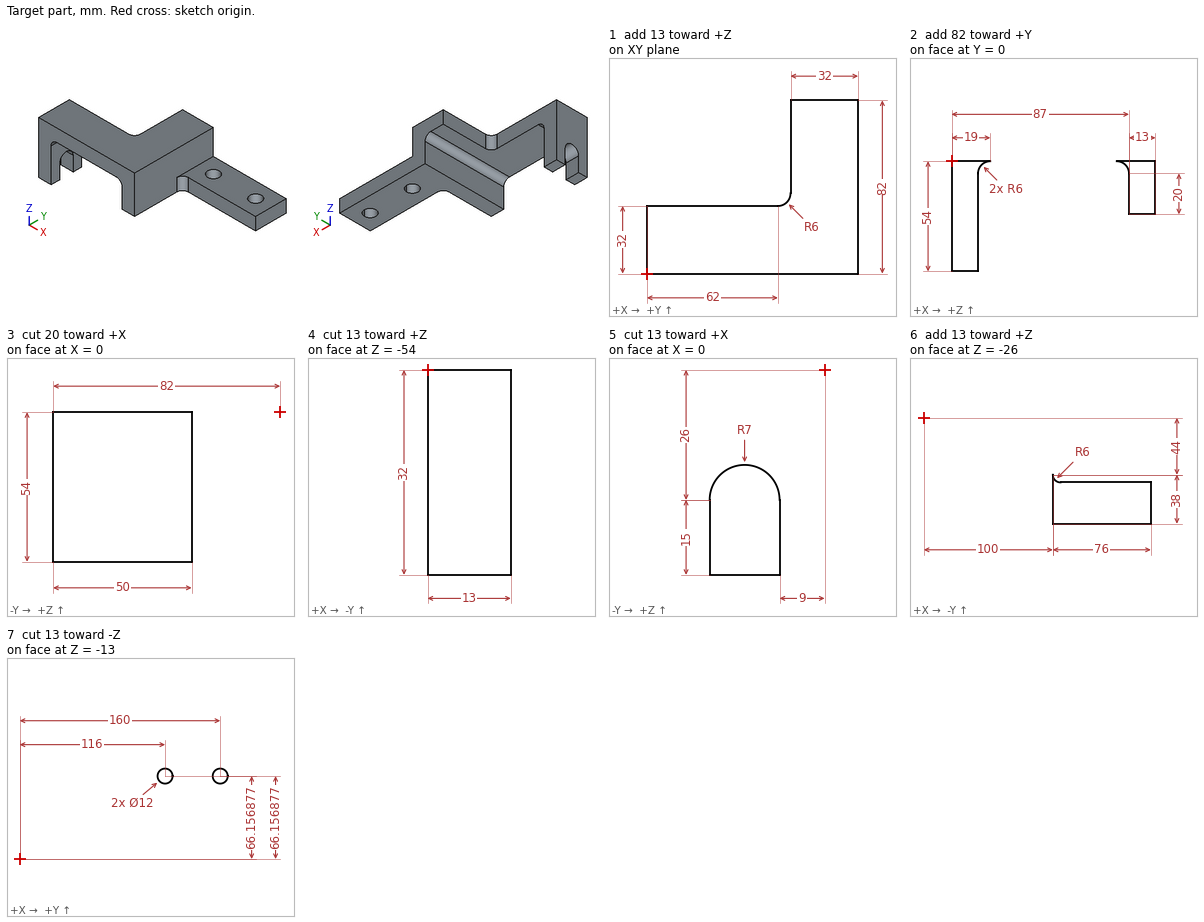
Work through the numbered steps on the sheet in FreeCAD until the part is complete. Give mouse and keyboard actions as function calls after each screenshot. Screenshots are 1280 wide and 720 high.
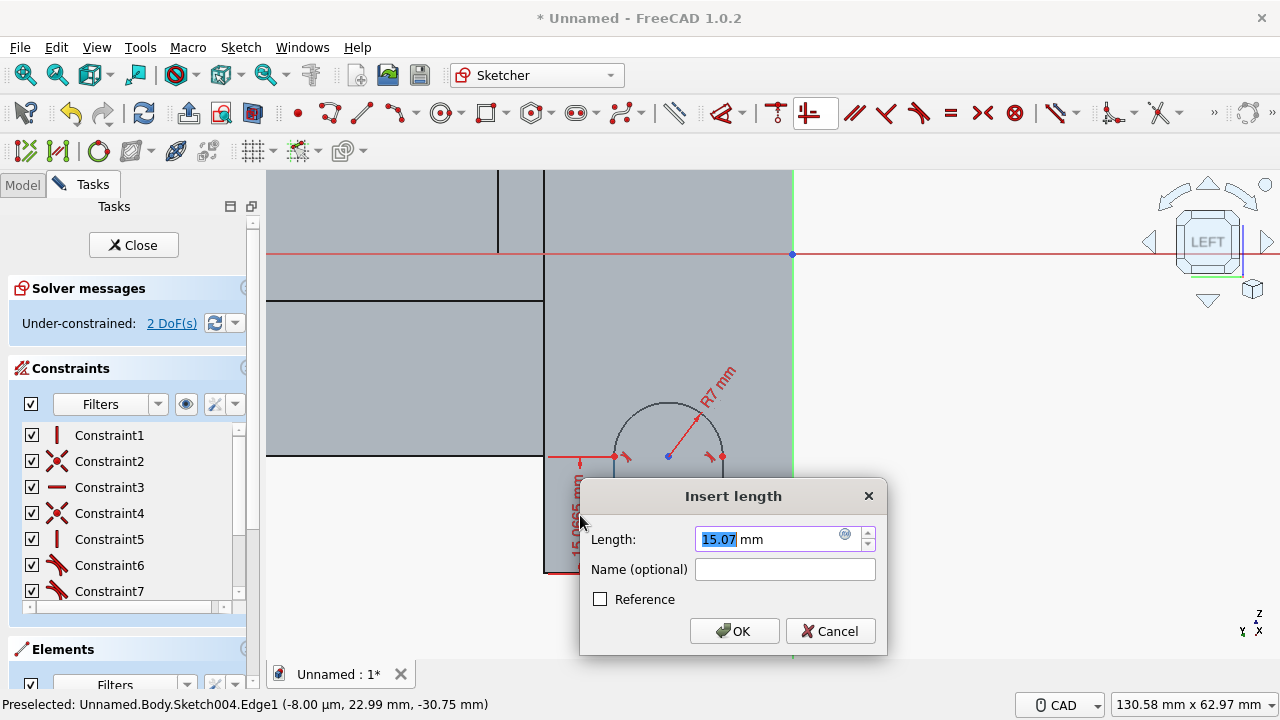
text(15)
key(Return)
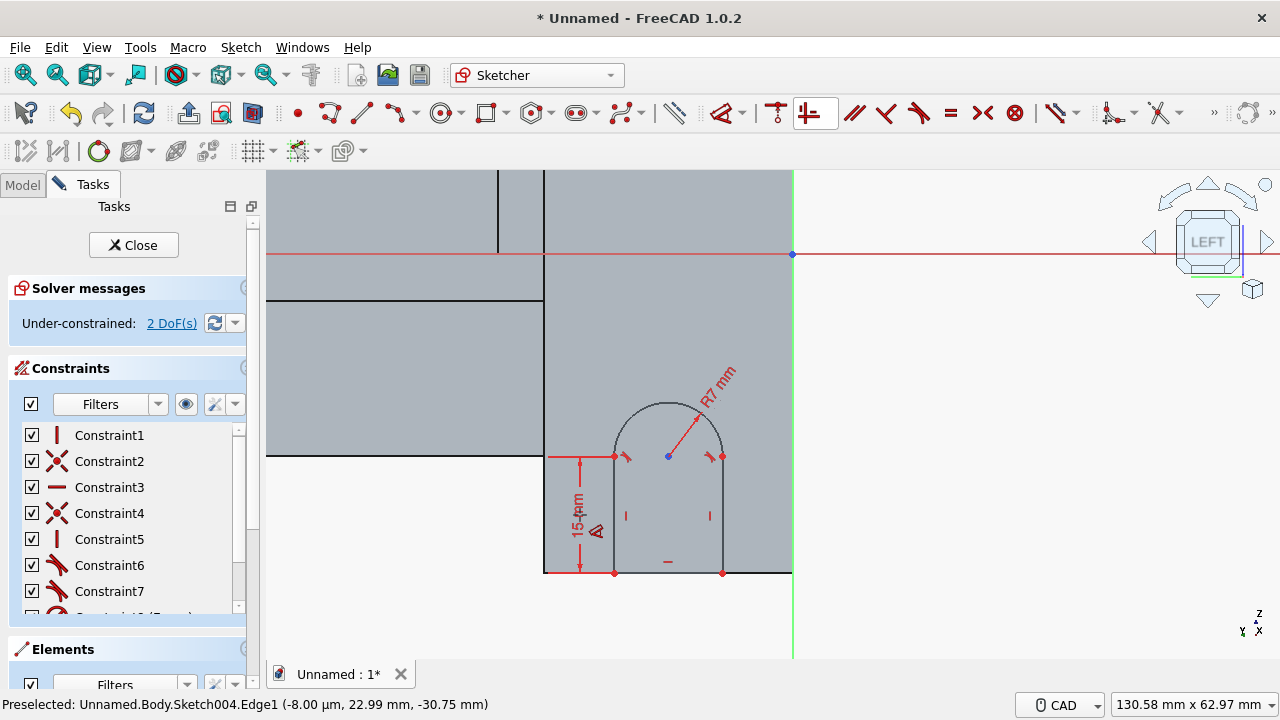
click(723, 573)
click(758, 607)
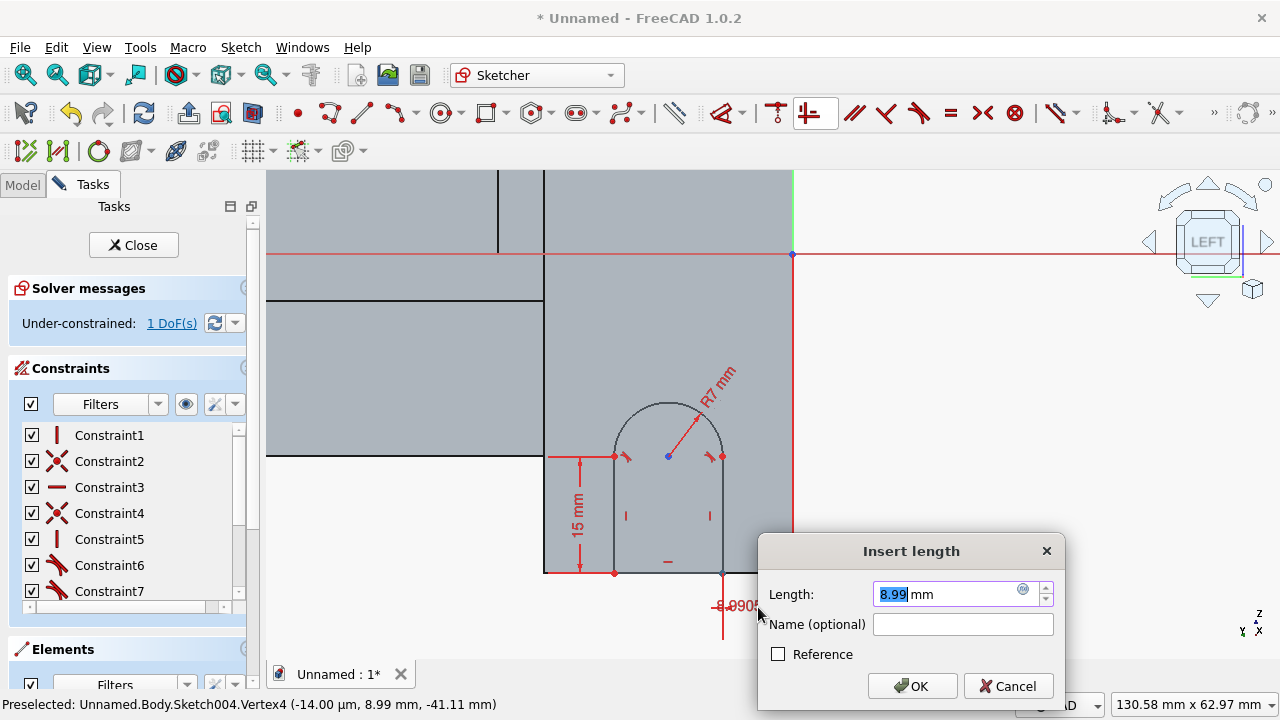
text(9)
key(Return)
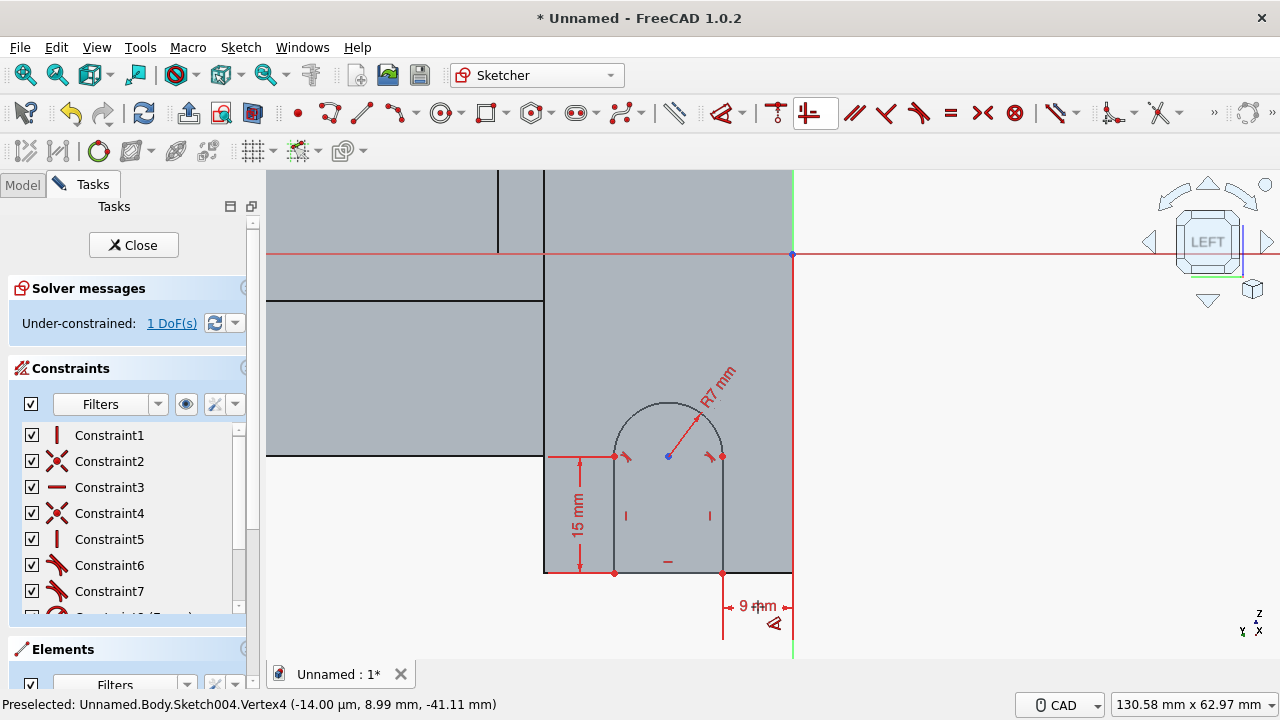
click(614, 457)
click(827, 356)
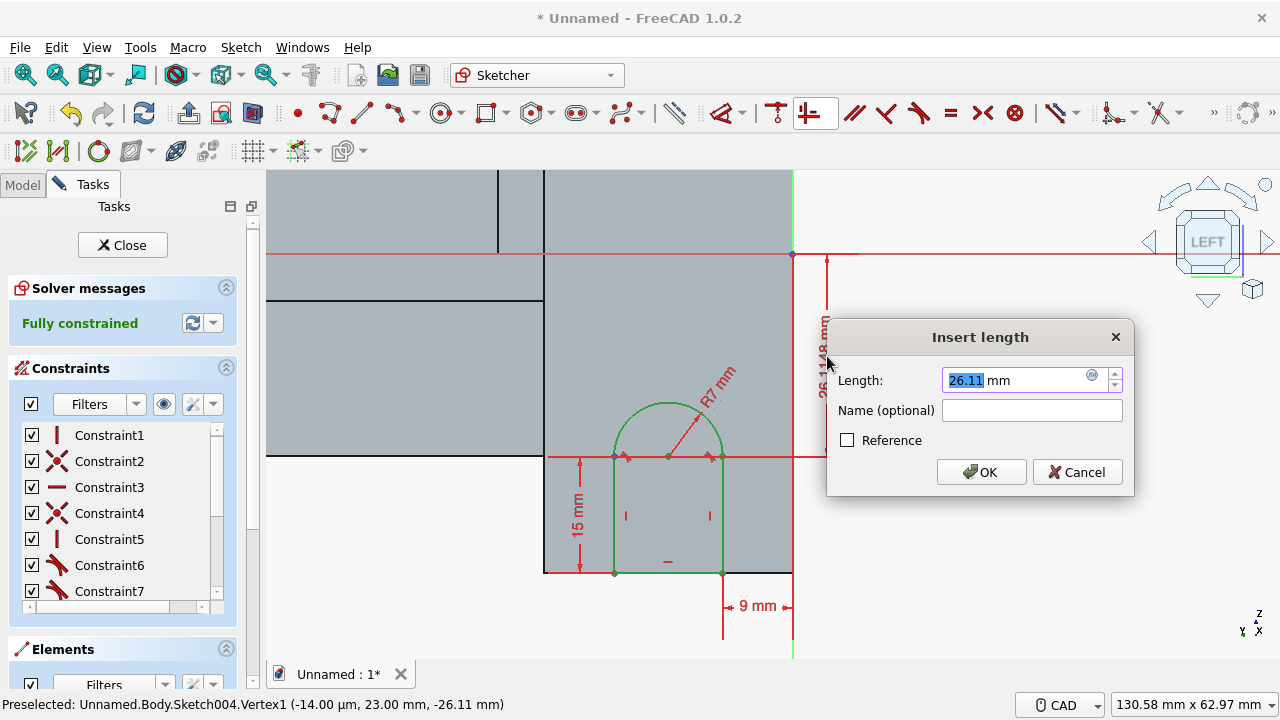
text(26)
key(Return)
key(Escape)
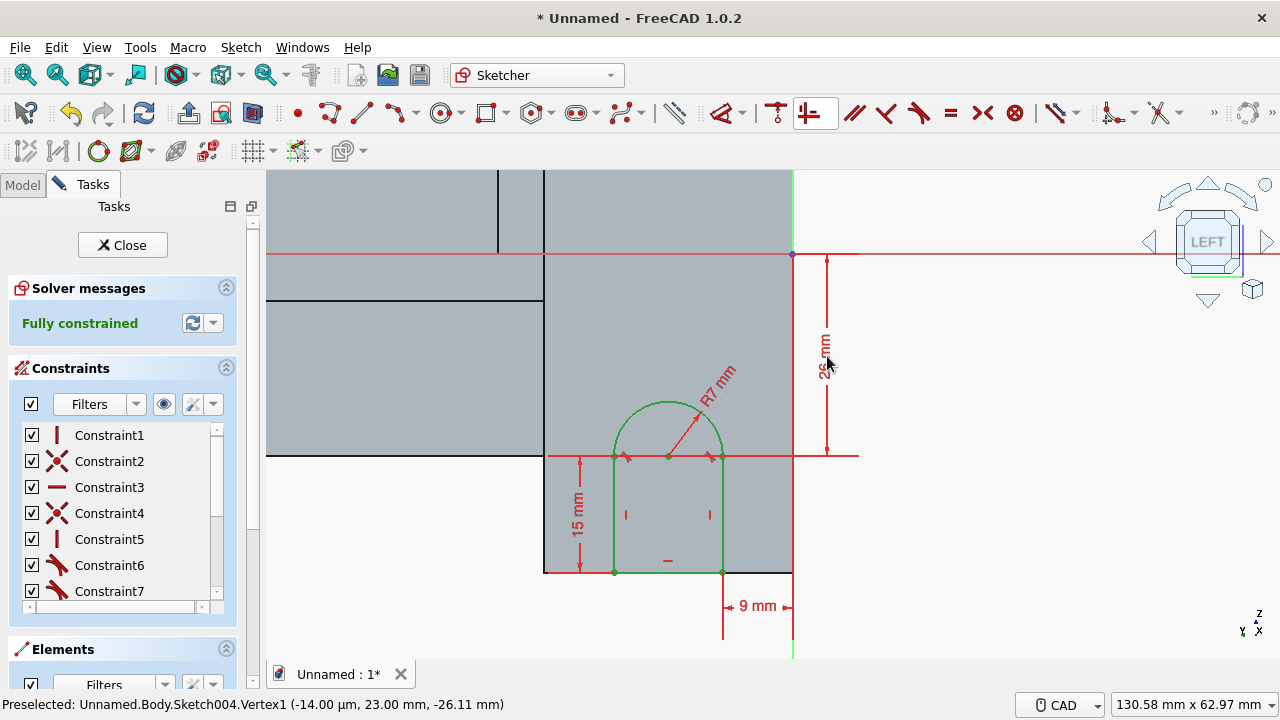
click(123, 245)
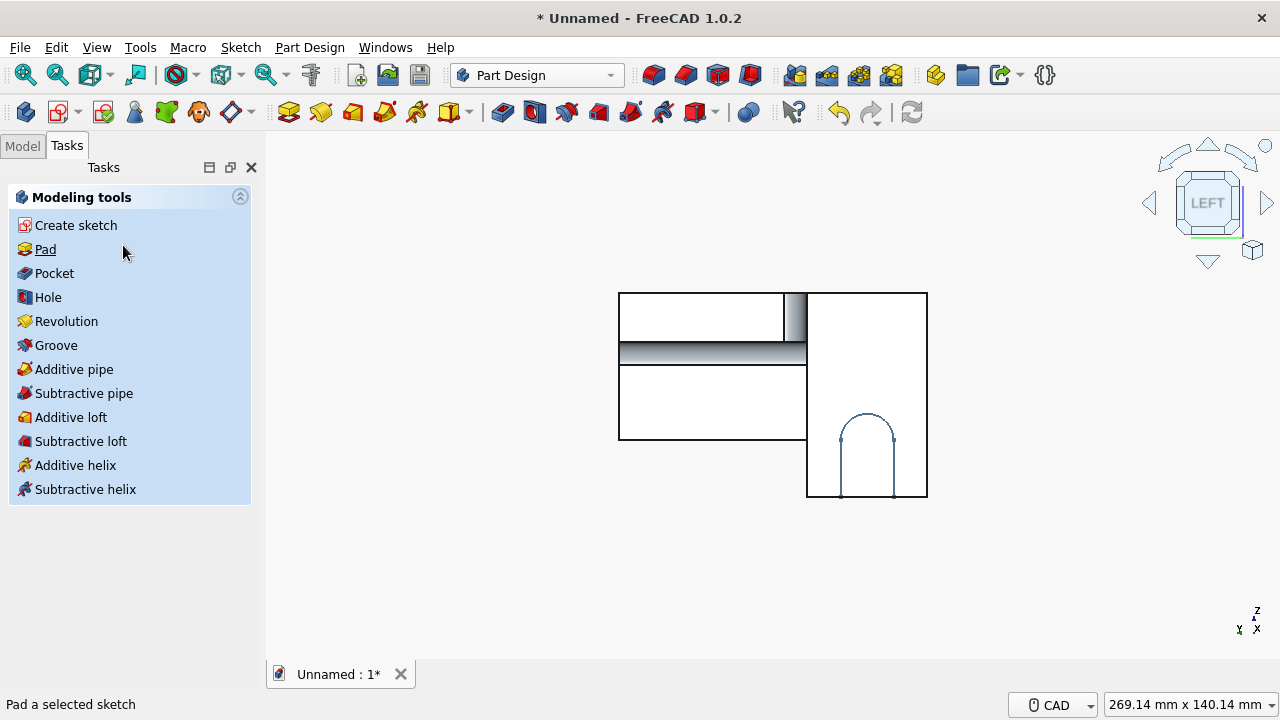
click(504, 112)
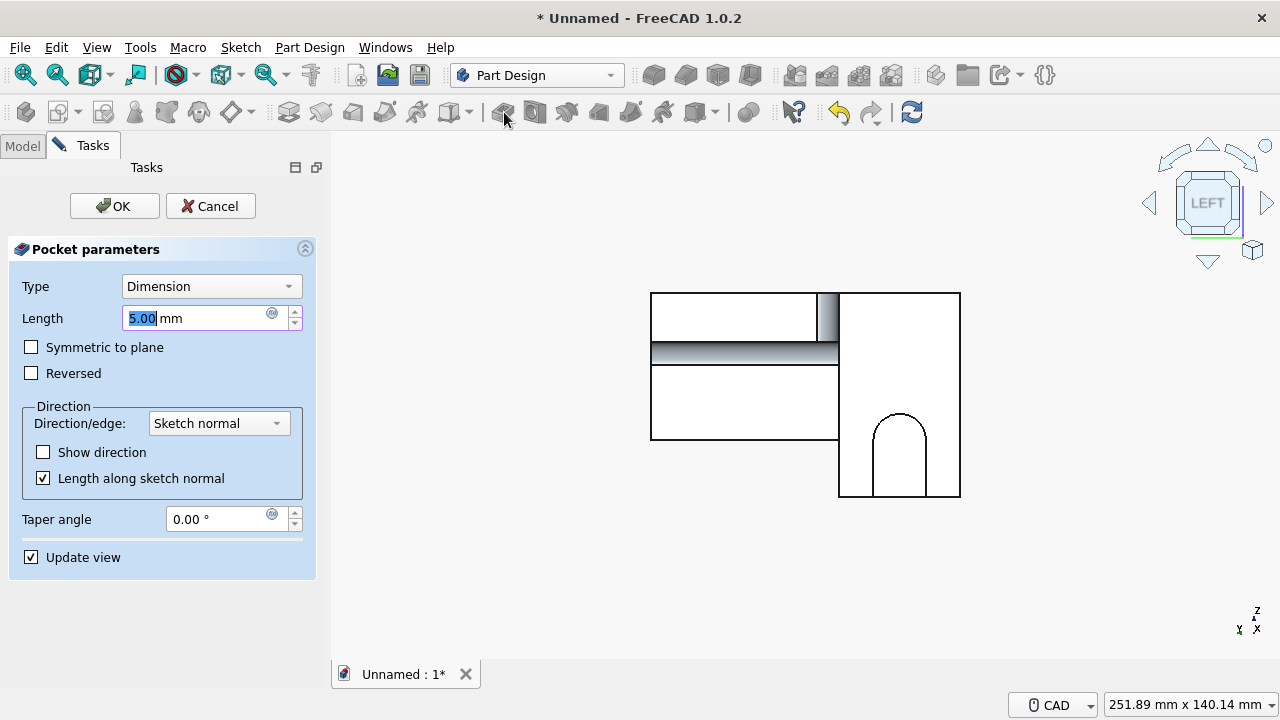
text(13)
key(Tab)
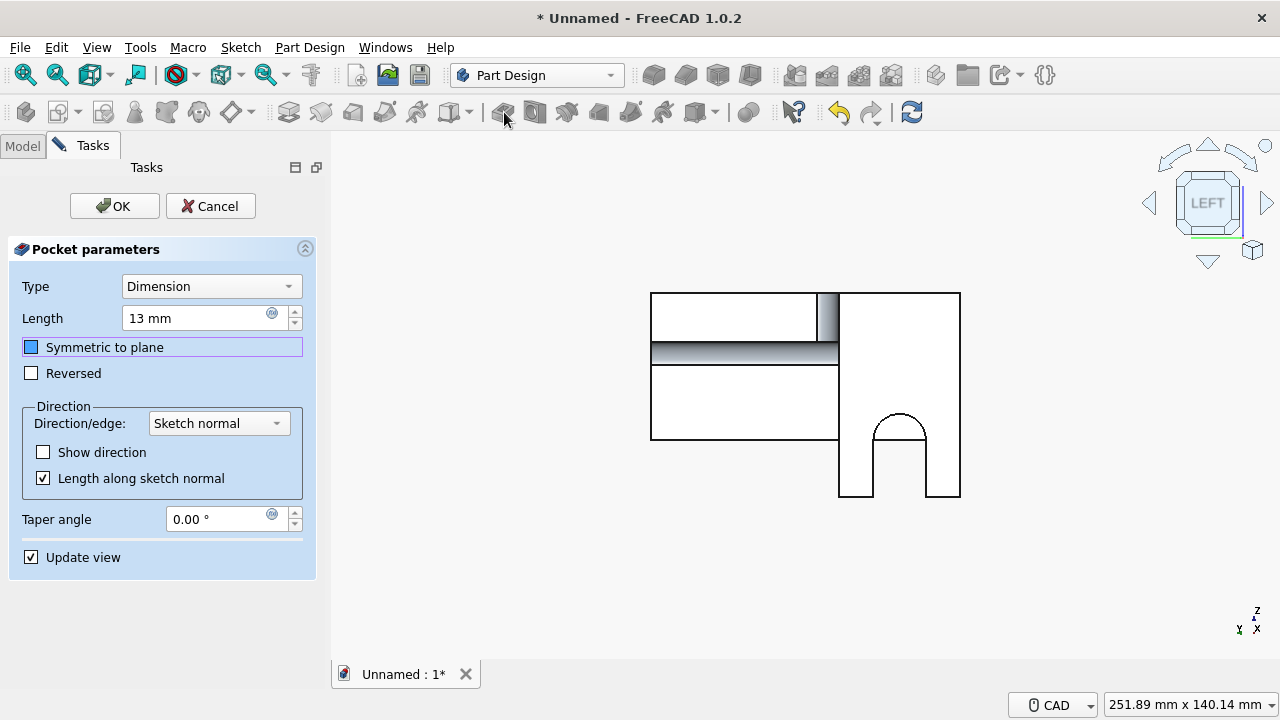
click(115, 206)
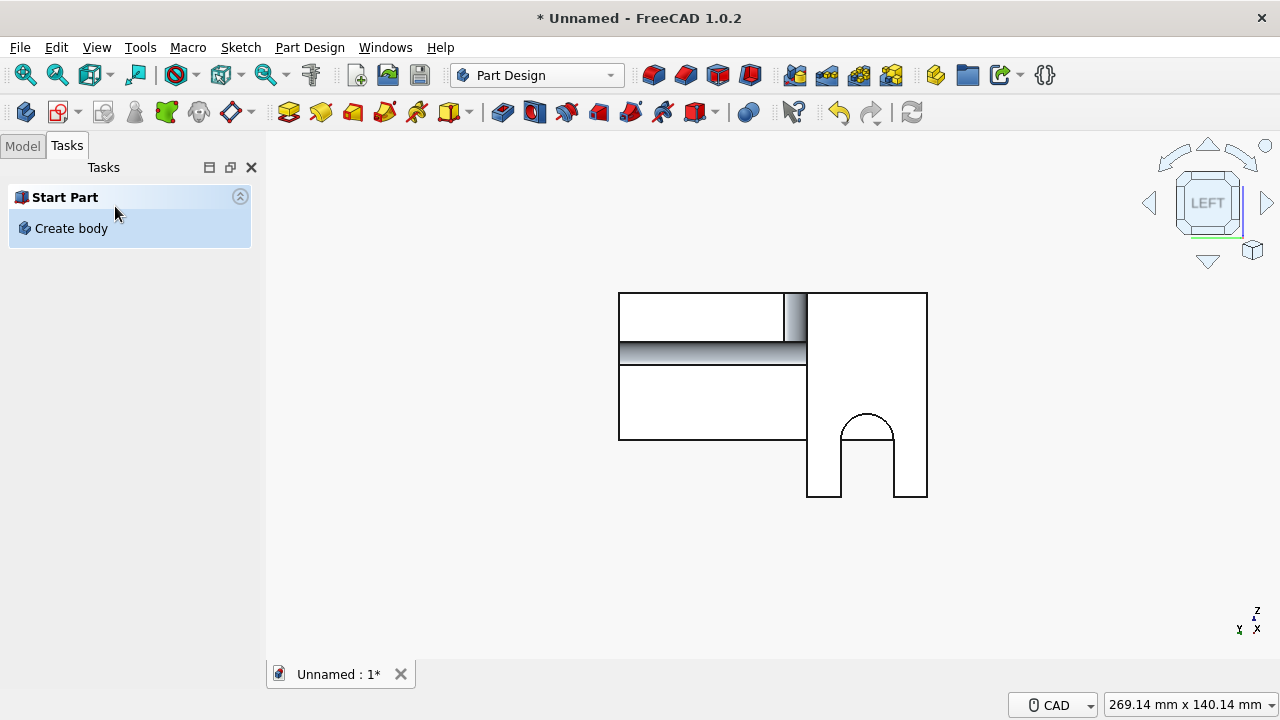
click(26, 76)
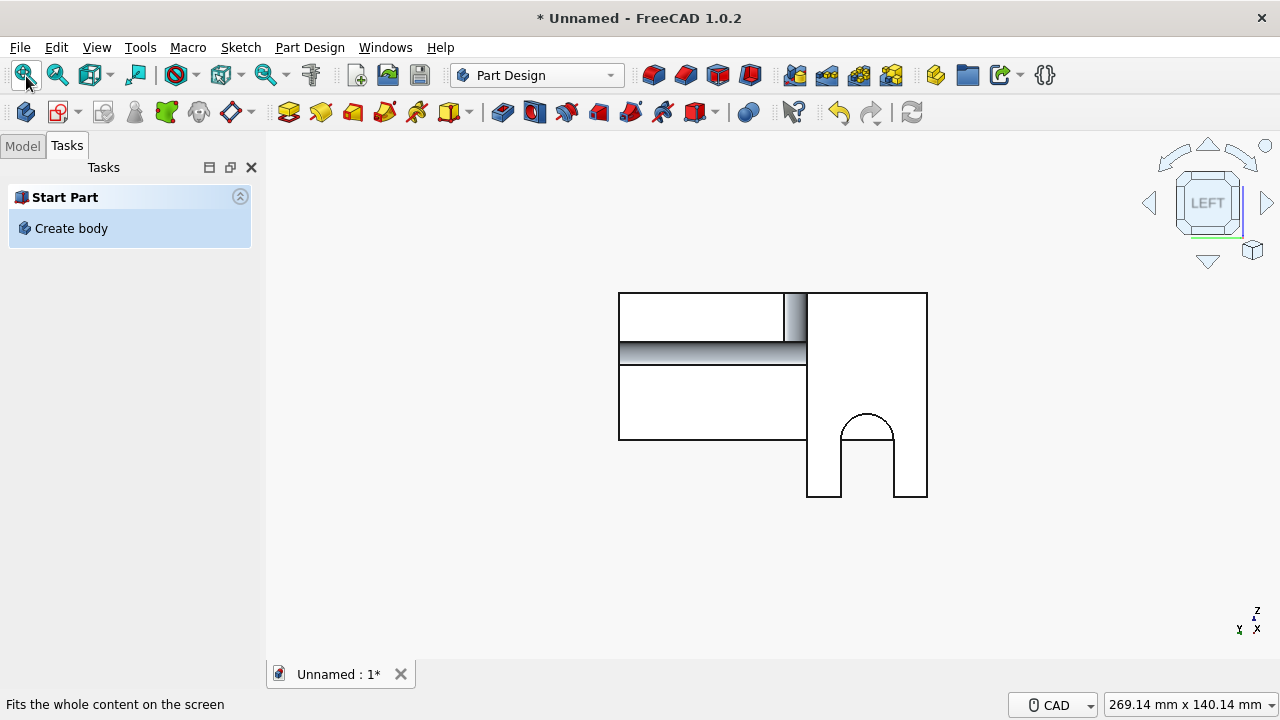
key(5)